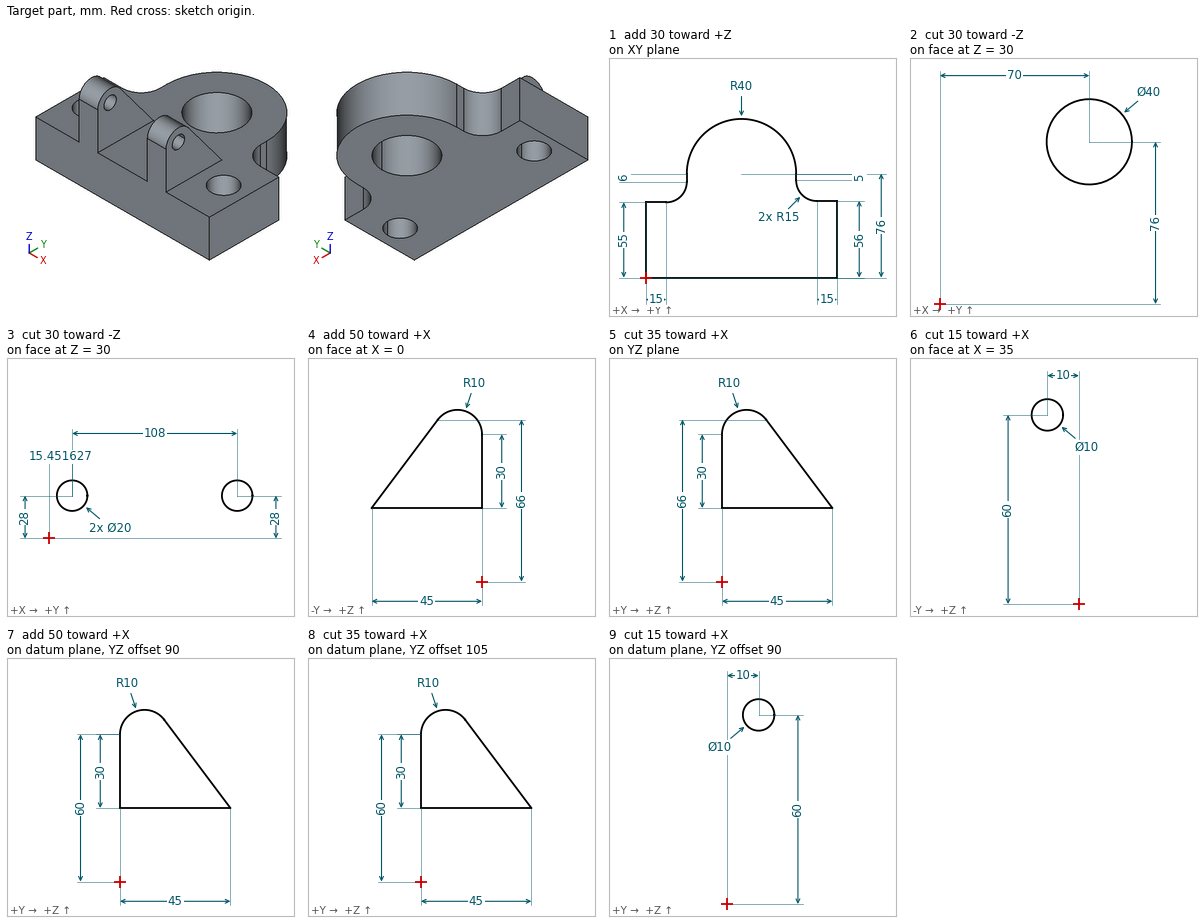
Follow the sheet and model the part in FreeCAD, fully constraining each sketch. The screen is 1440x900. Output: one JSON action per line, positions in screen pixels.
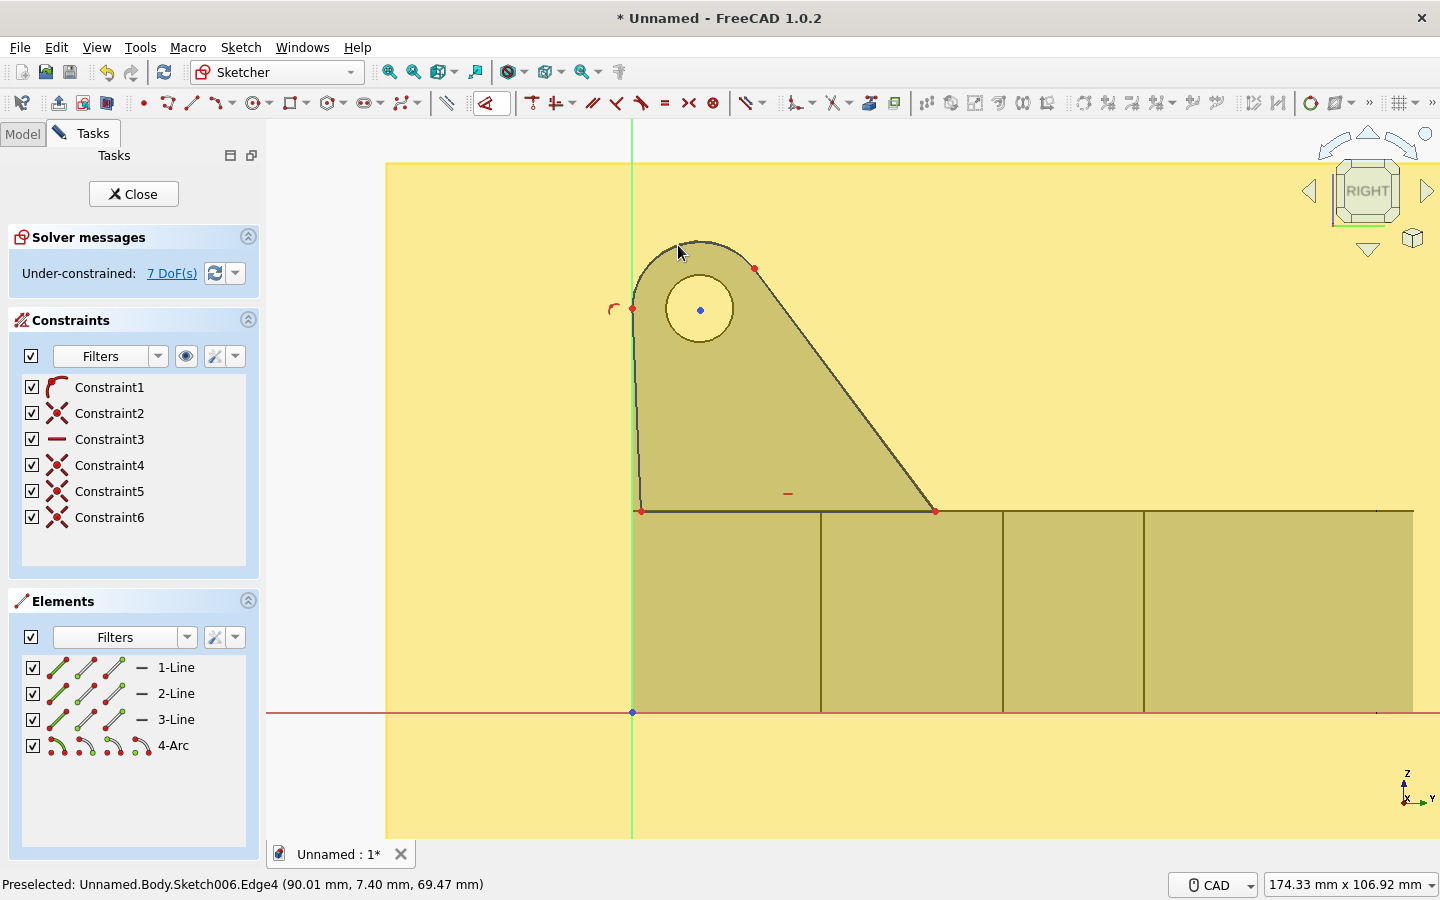
{"action": "left_click", "coordinate": [635, 370]}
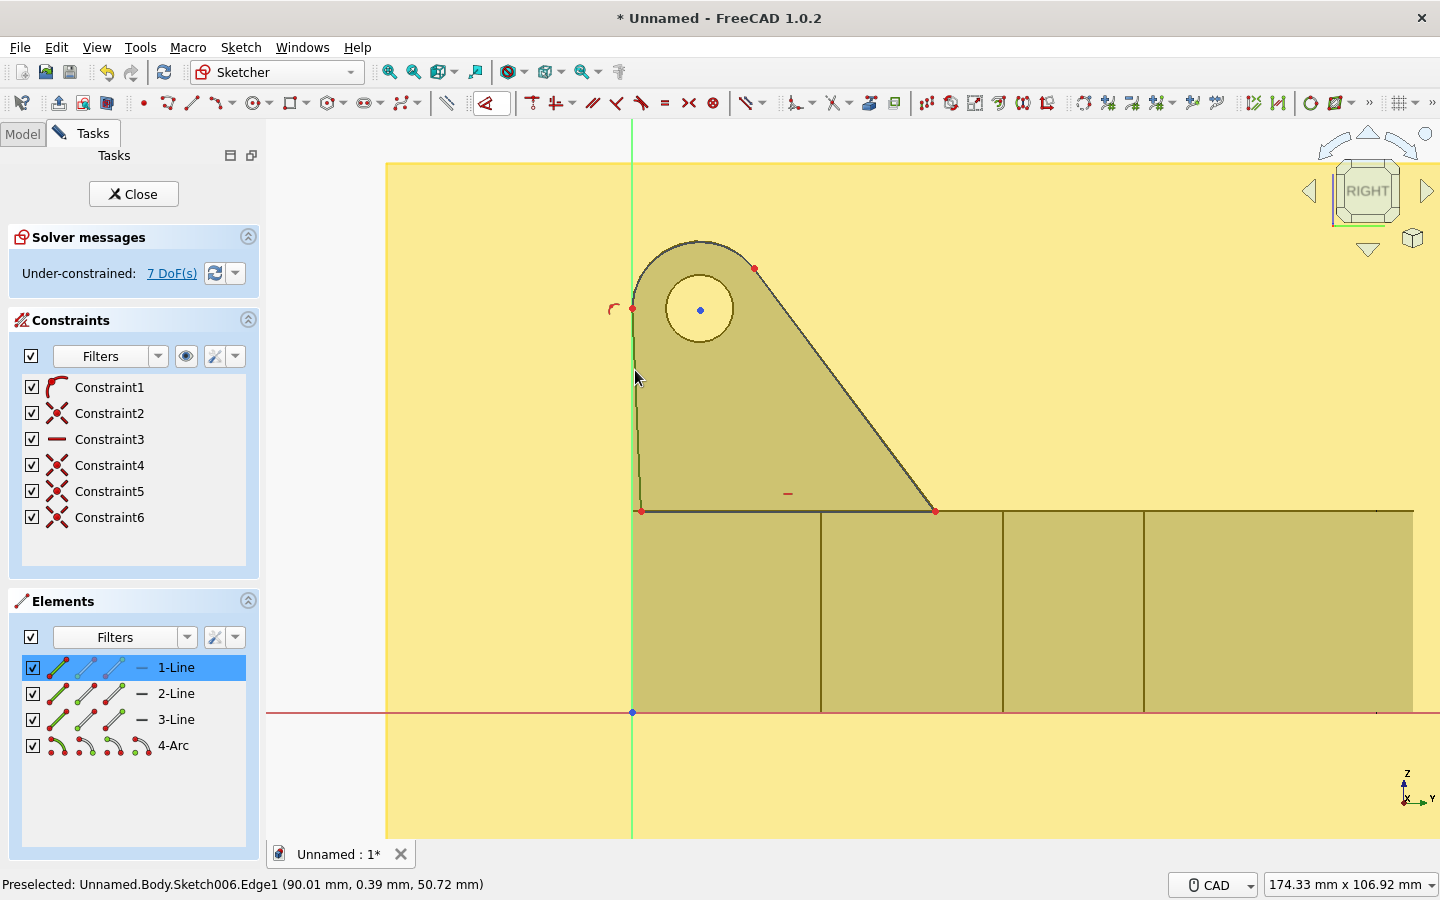
{"action": "left_click", "coordinate": [712, 243]}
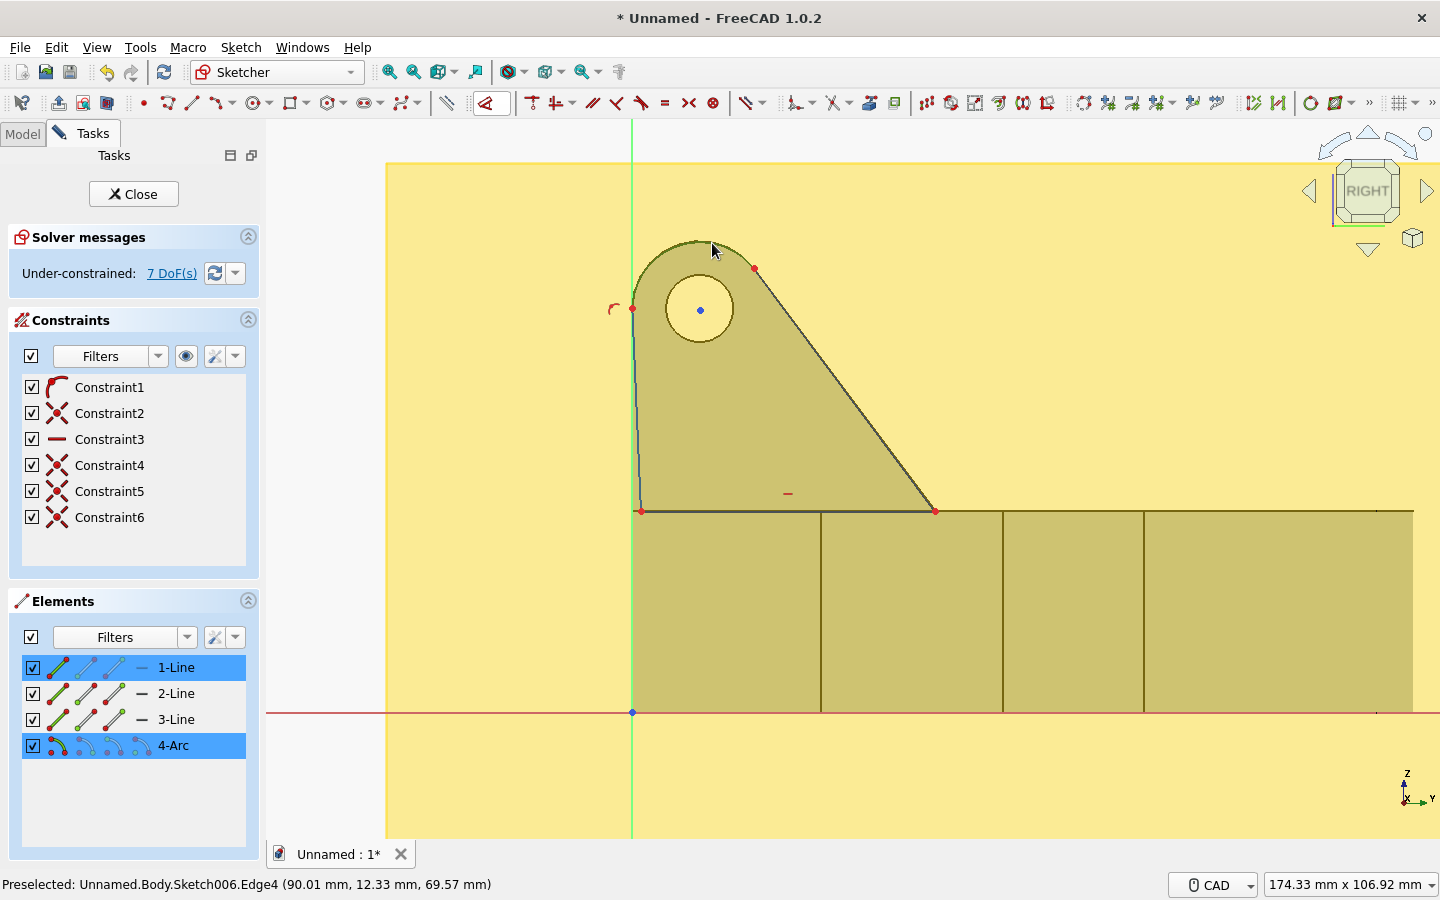
{"action": "key", "text": "t"}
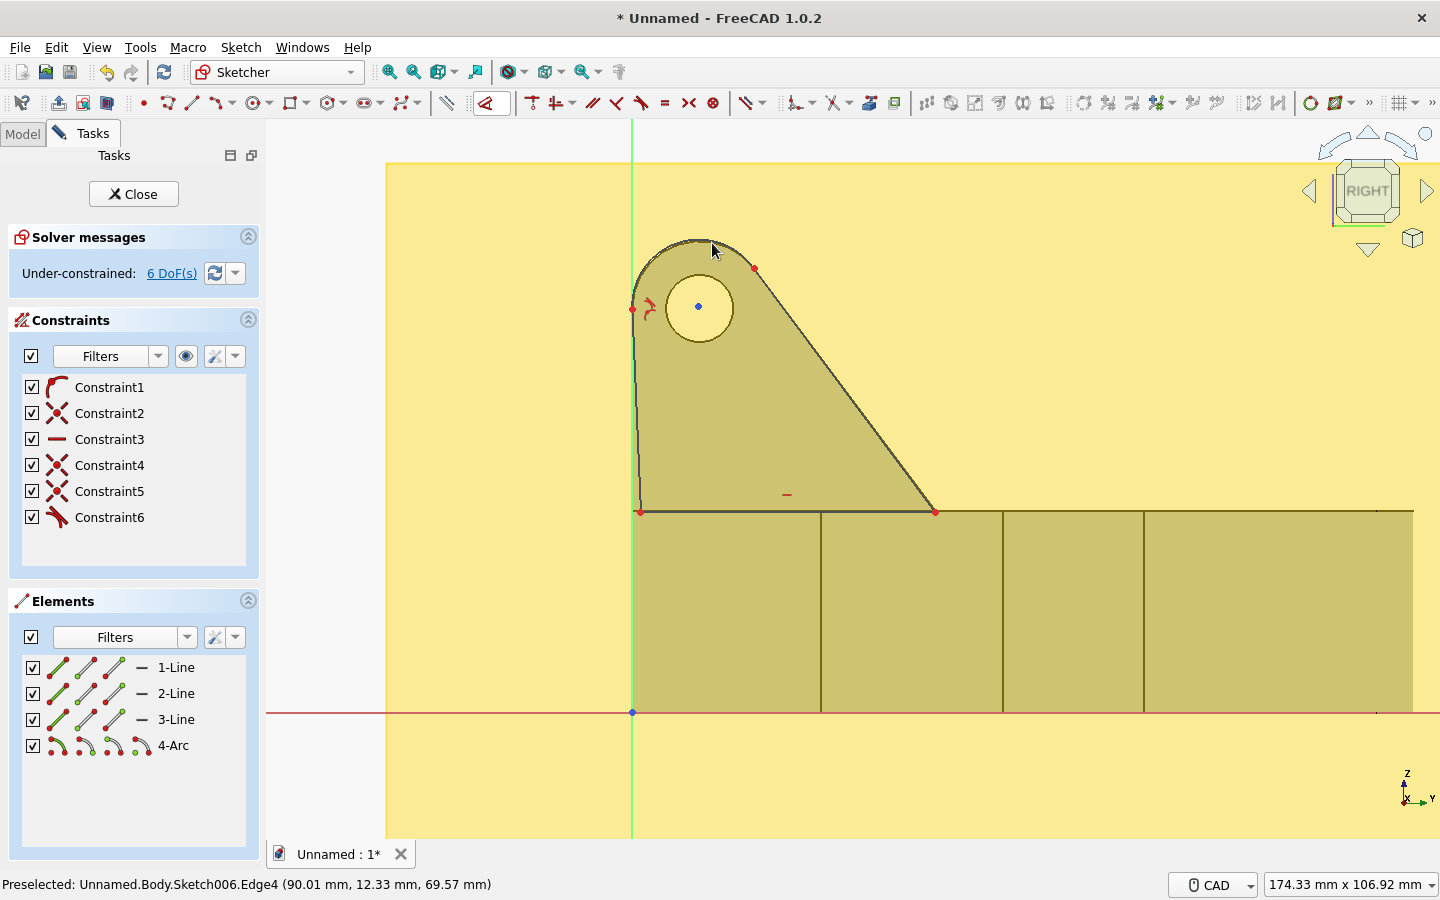
{"action": "left_click", "coordinate": [881, 439]}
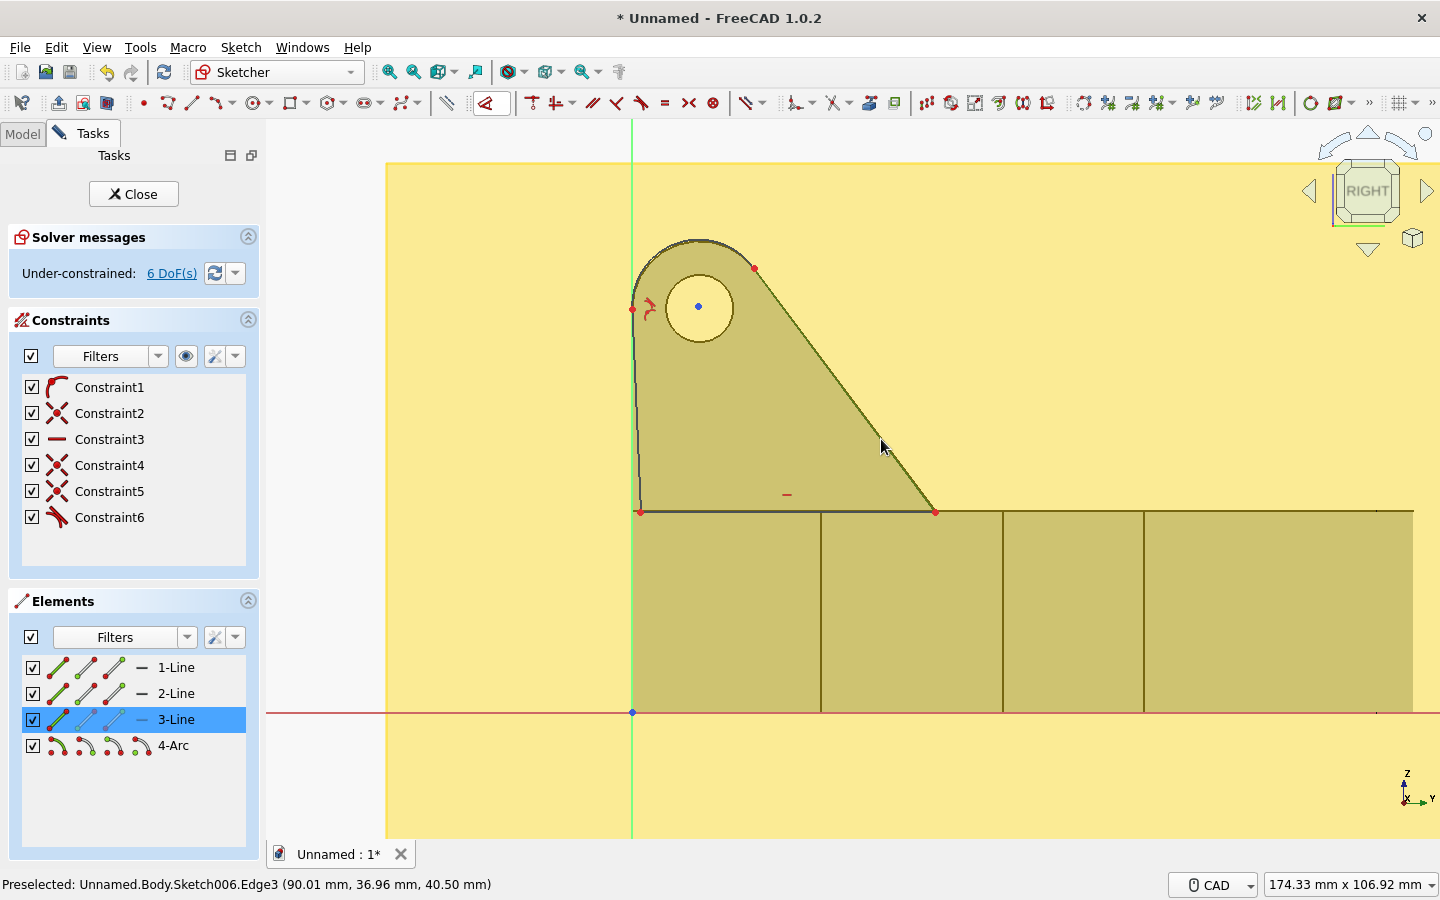
{"action": "left_click", "coordinate": [712, 241]}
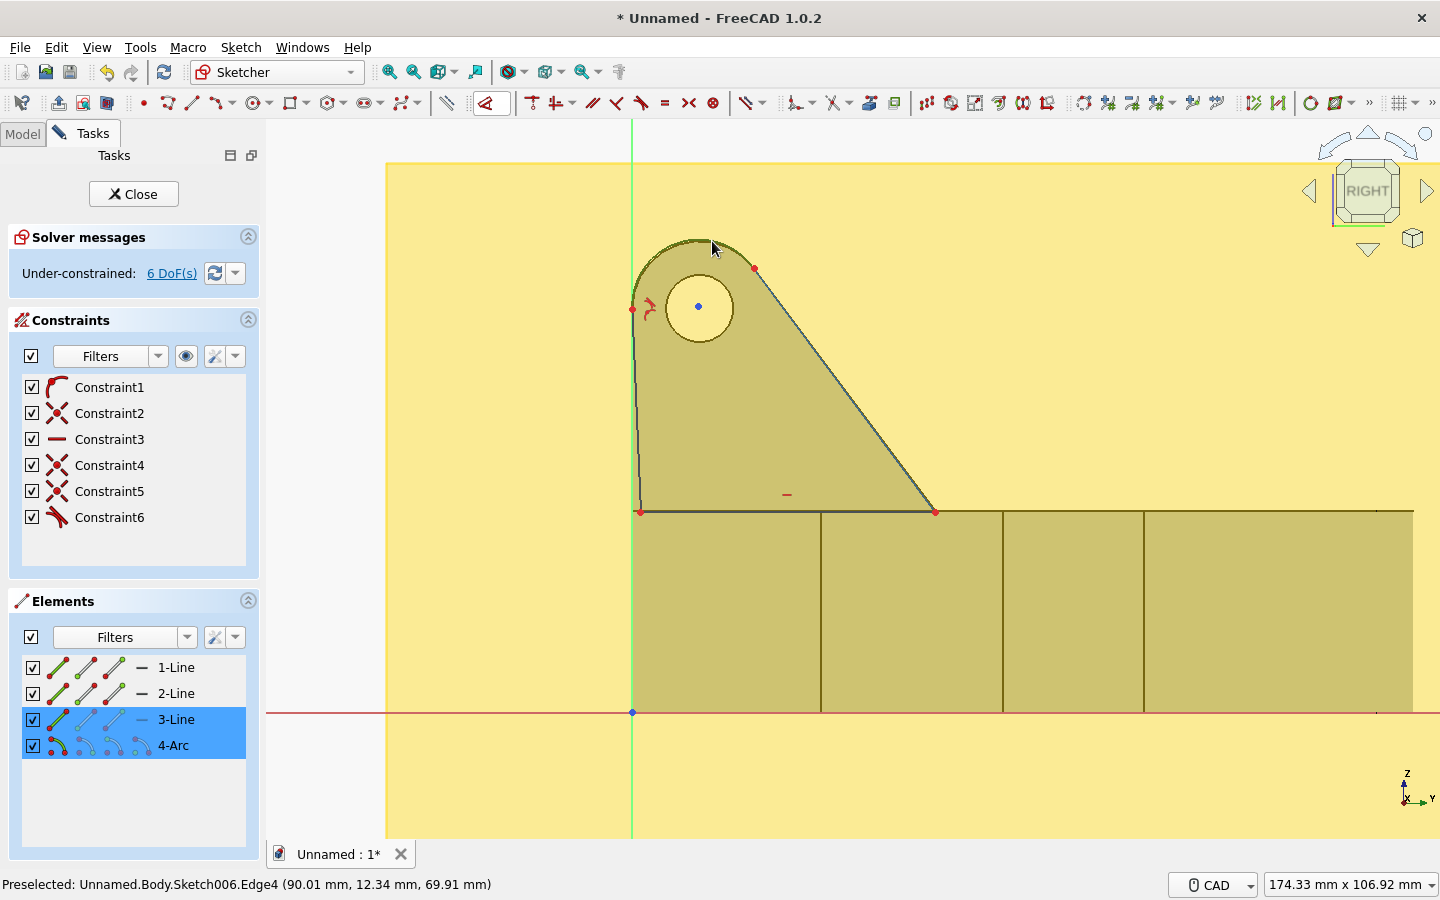
{"action": "key", "text": "t"}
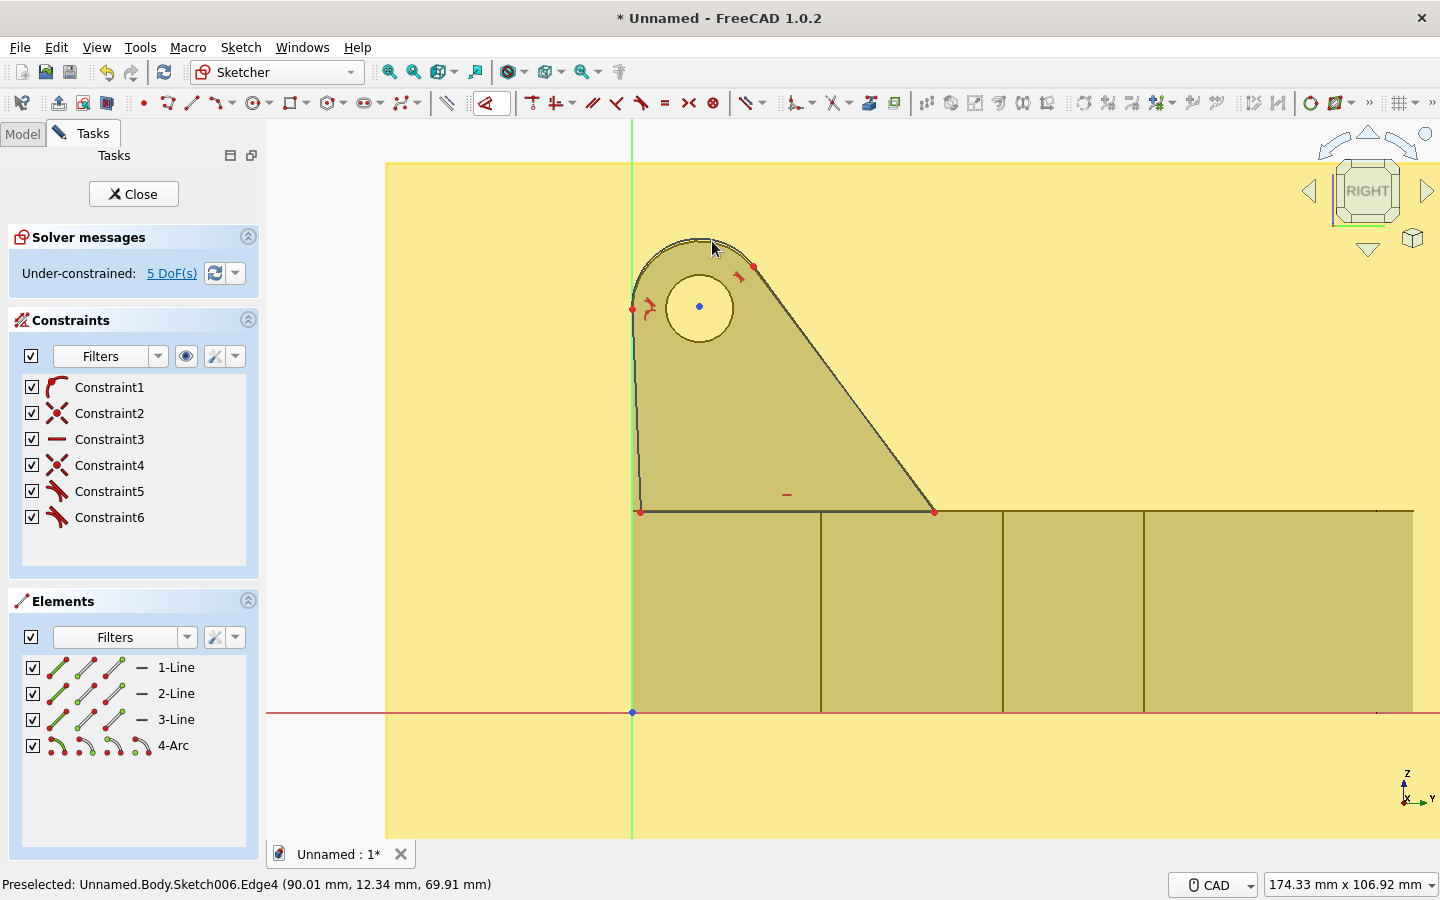
{"action": "left_click", "coordinate": [635, 370]}